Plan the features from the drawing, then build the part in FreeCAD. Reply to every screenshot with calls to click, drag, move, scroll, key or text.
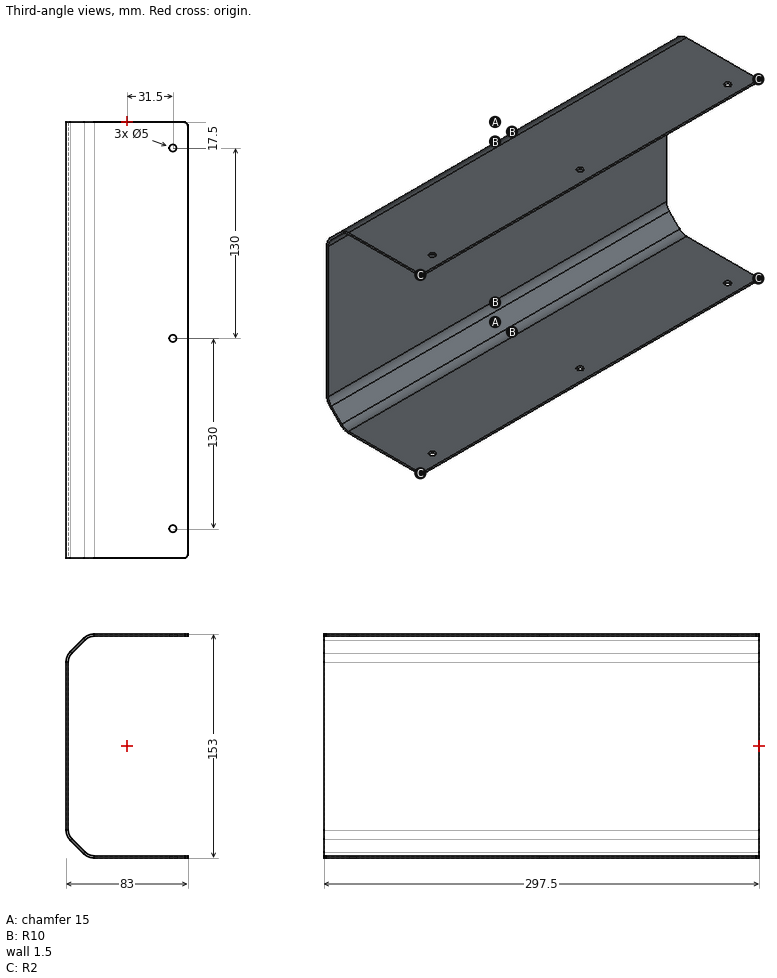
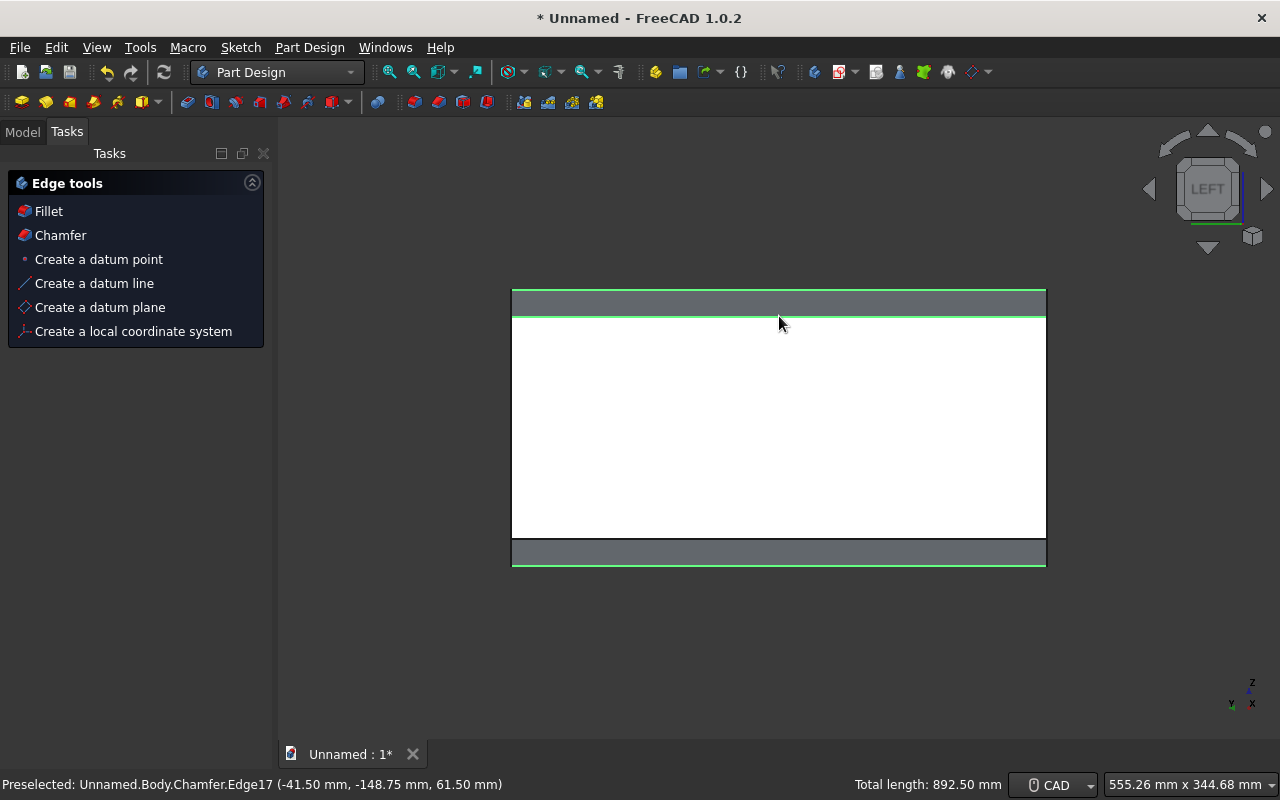
click(779, 538, ctrl)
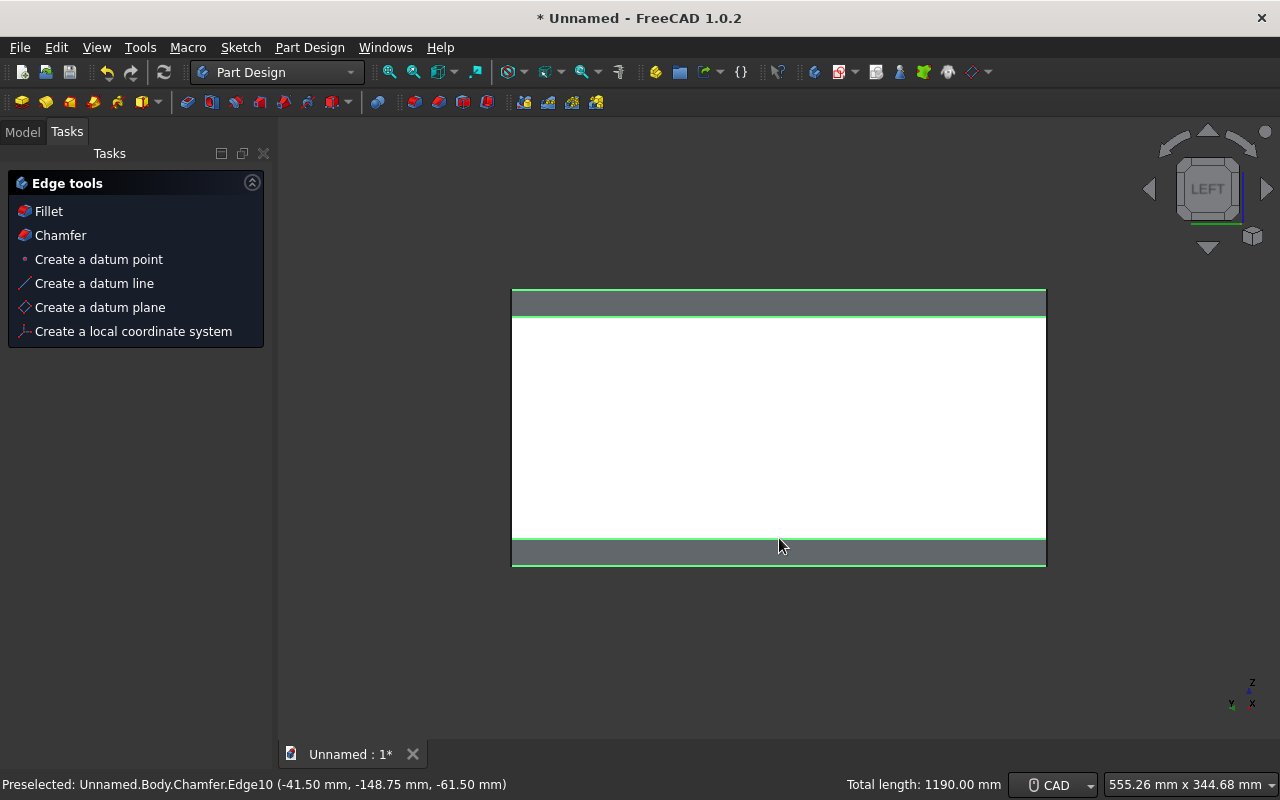
click(416, 102)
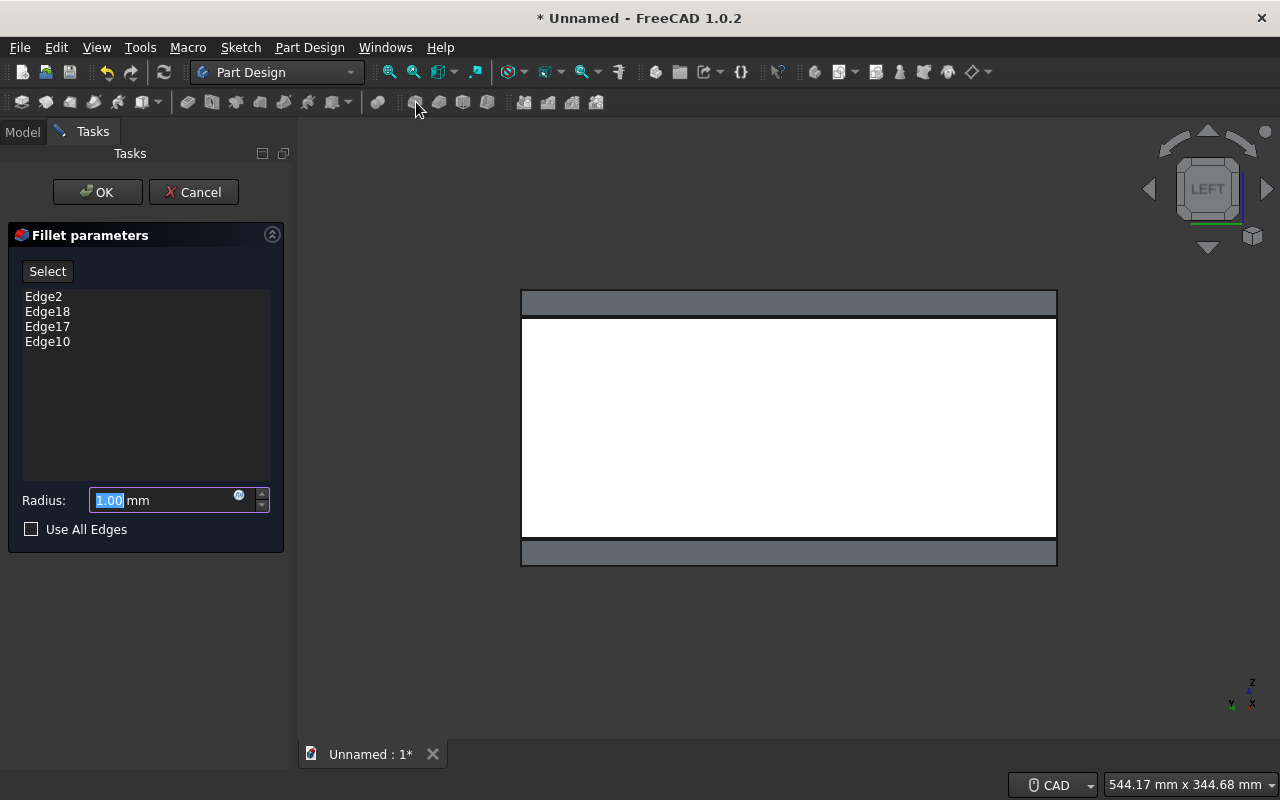
text(10)
key(Tab)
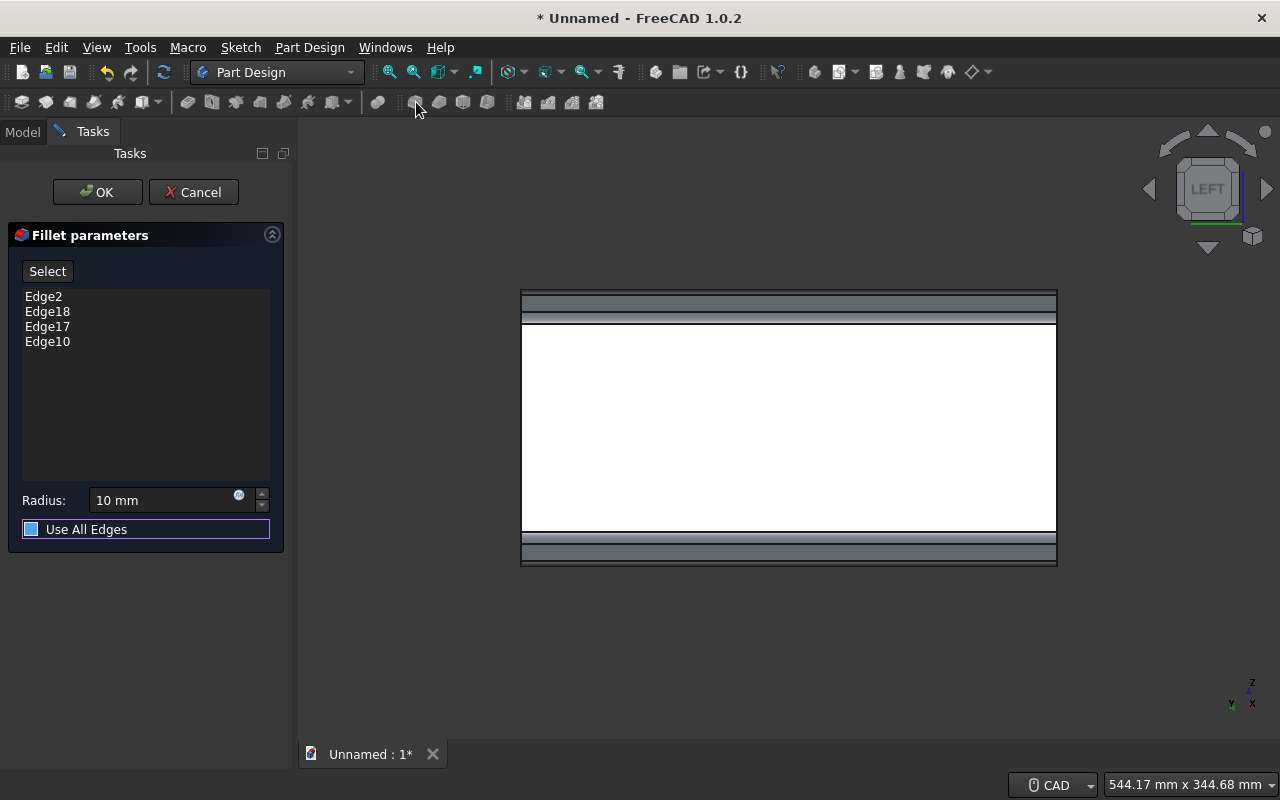
click(98, 192)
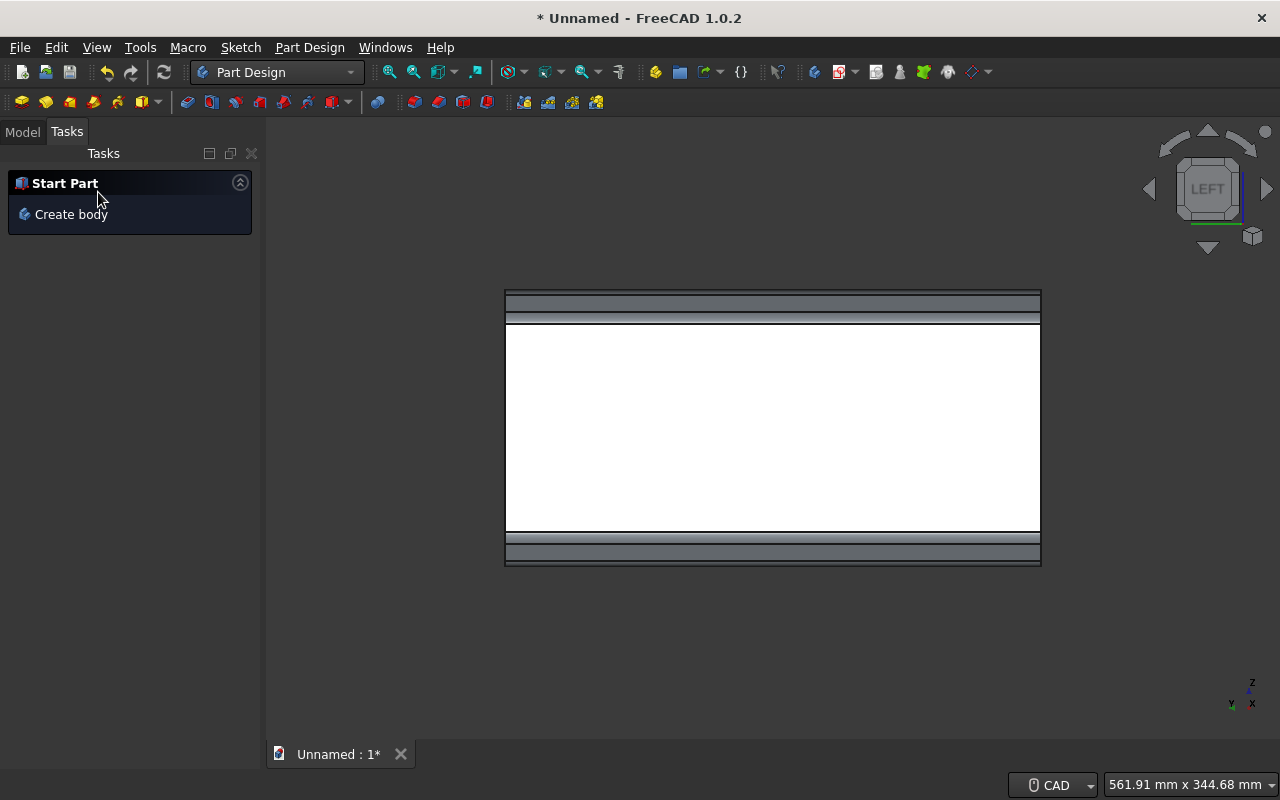
key(0)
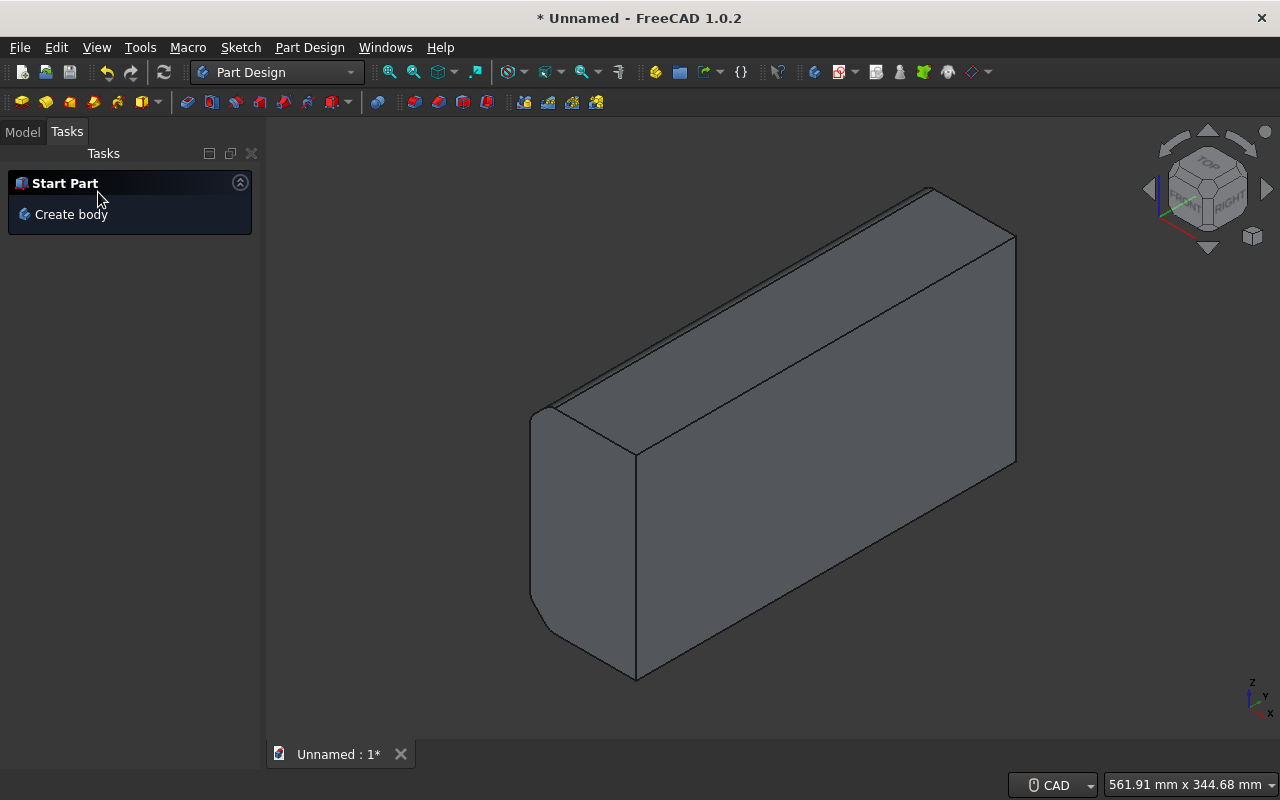
click(583, 504)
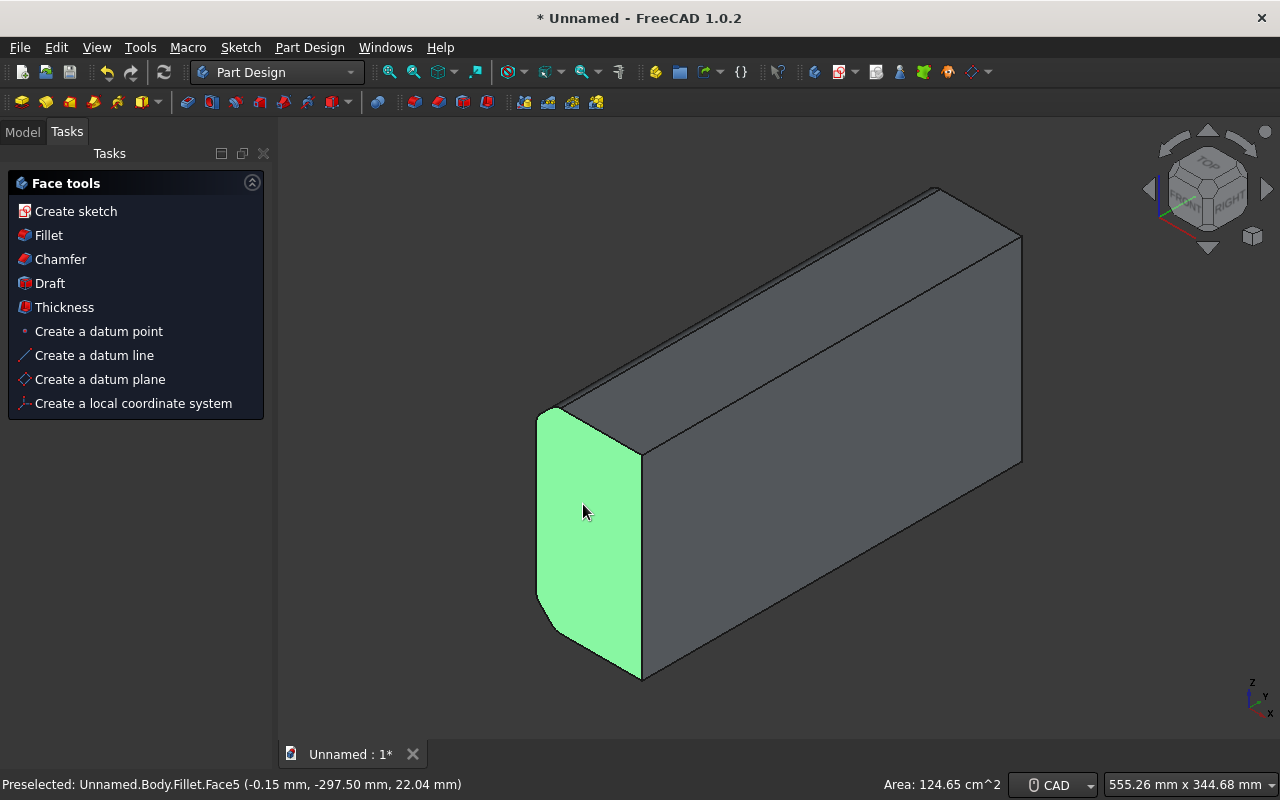
click(778, 489, ctrl)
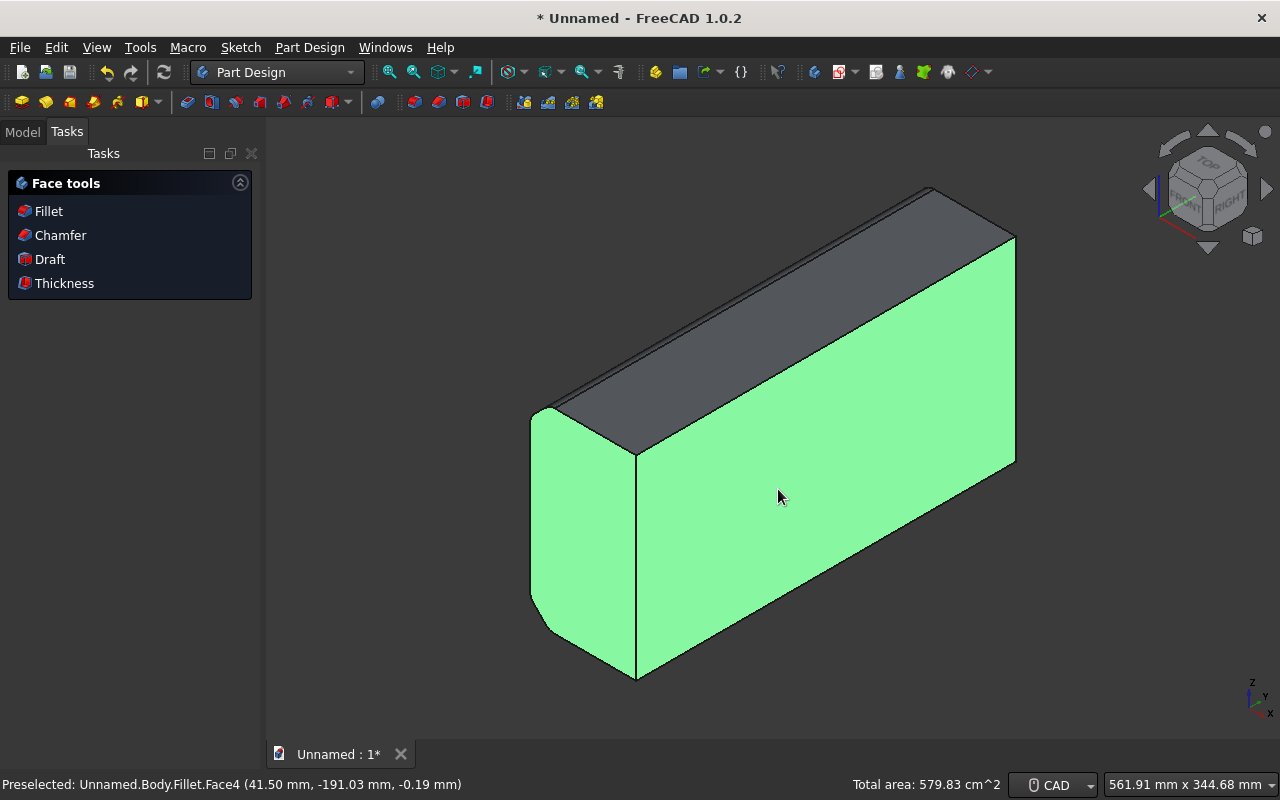
key(2)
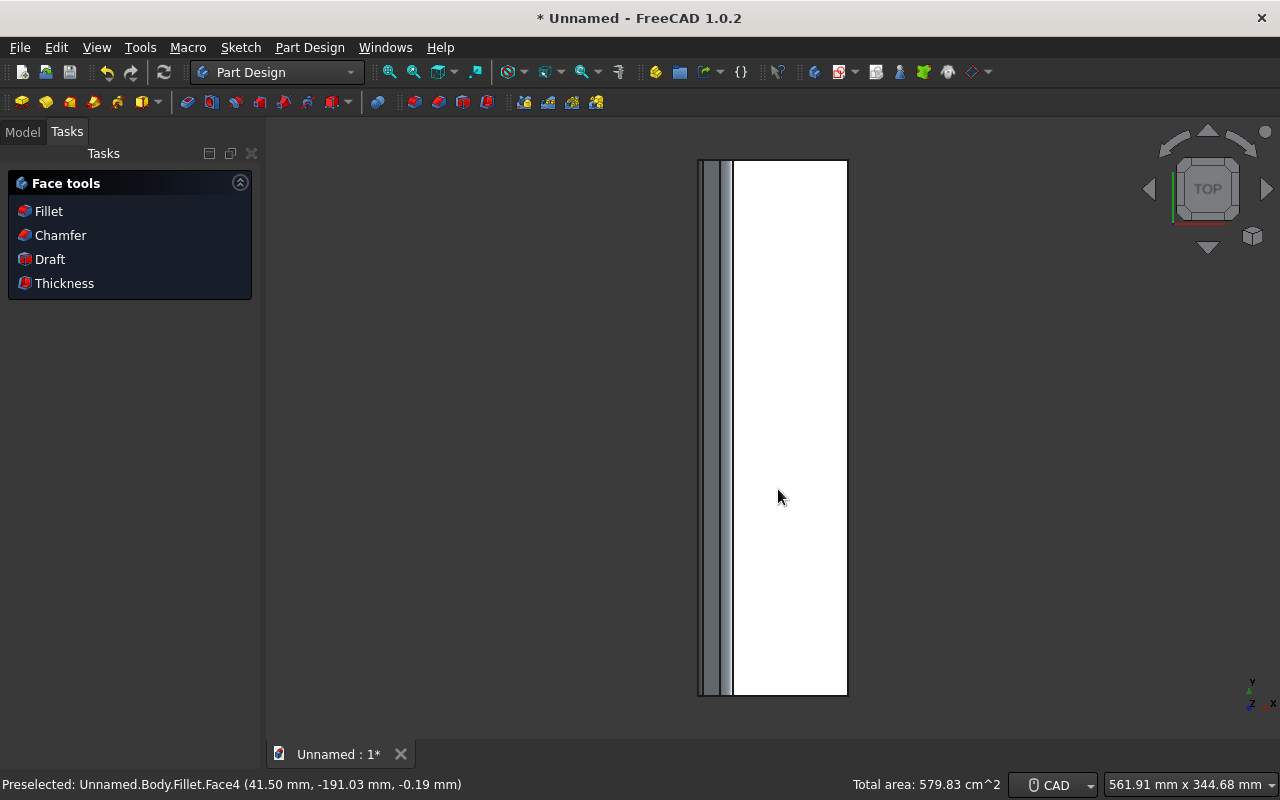
key(1)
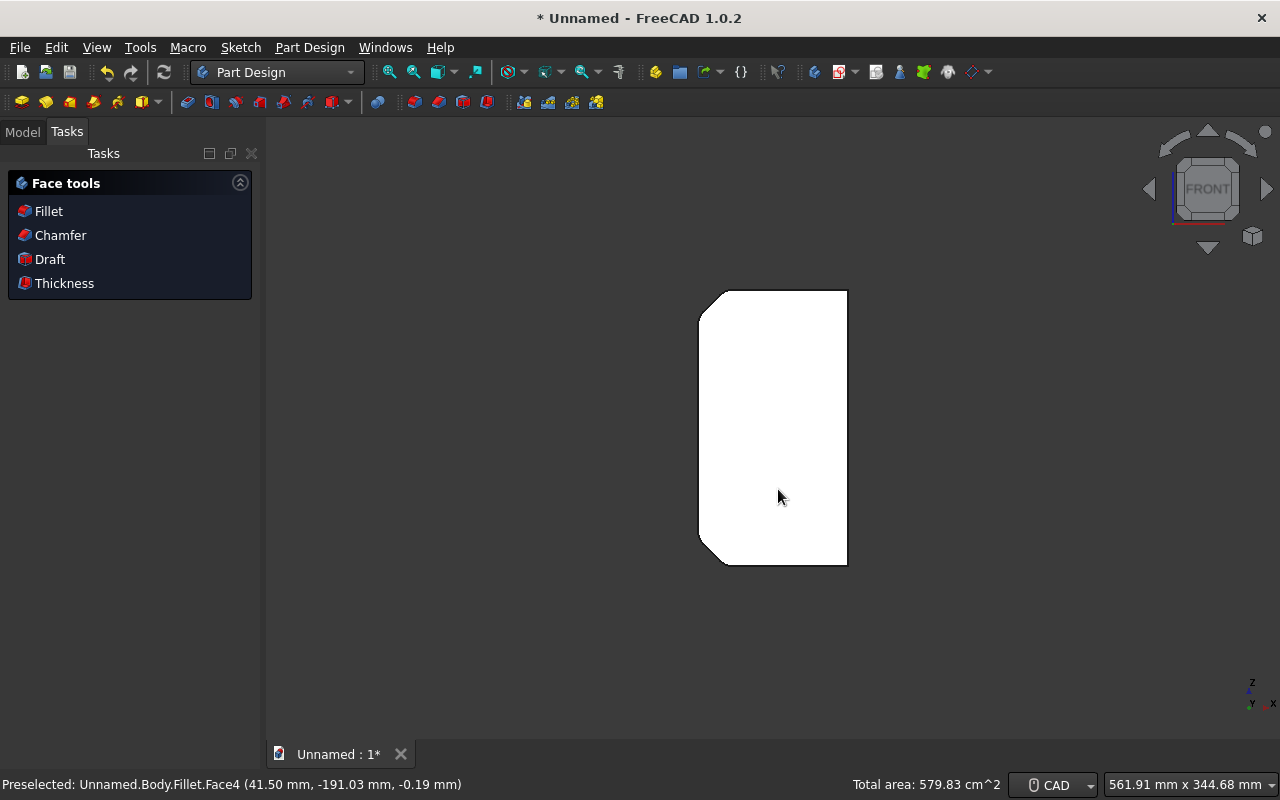
key(v)
key(f)